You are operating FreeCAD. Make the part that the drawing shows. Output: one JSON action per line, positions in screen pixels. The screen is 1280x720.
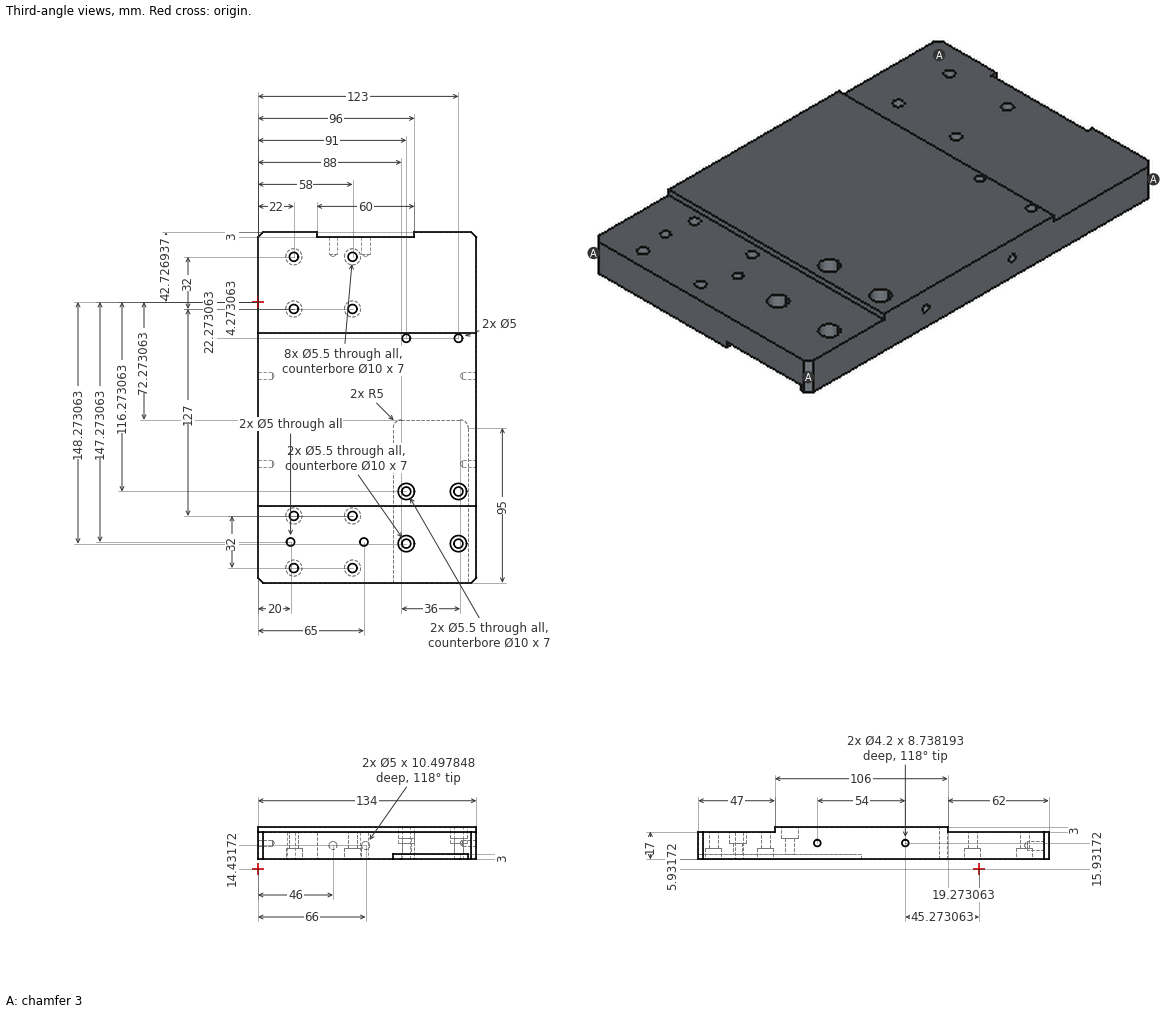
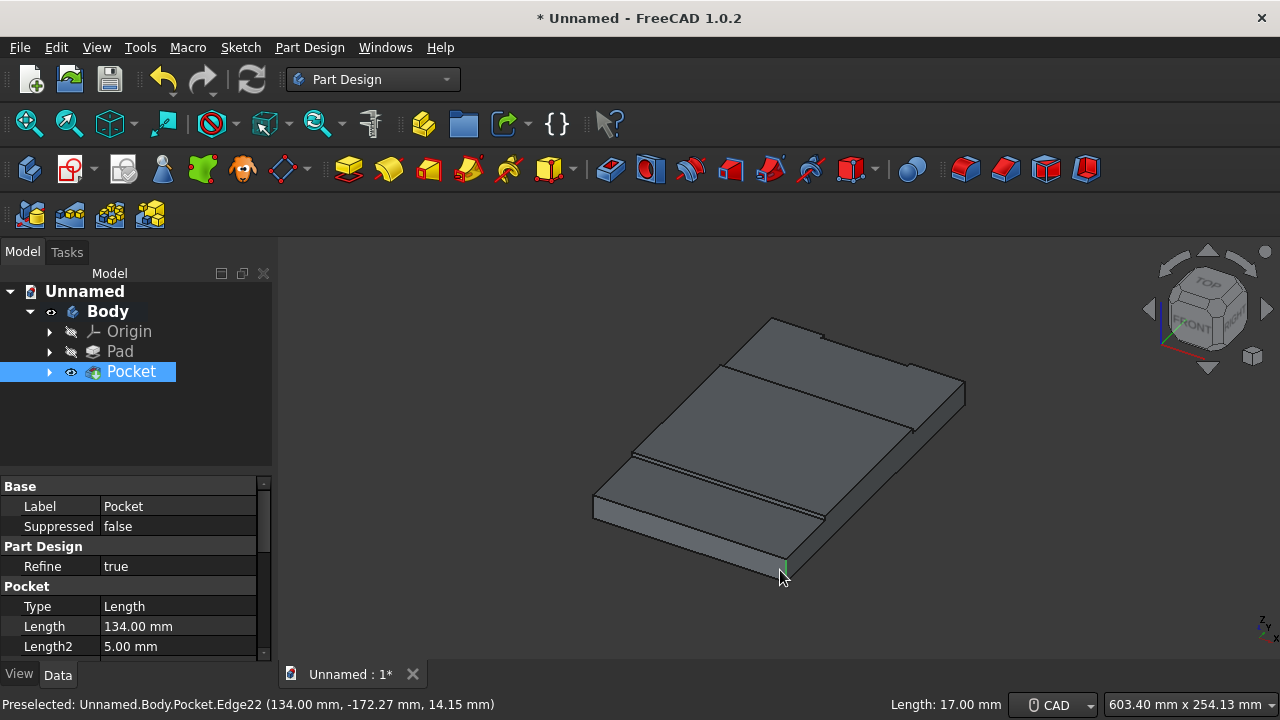
{"action": "key", "text": "0"}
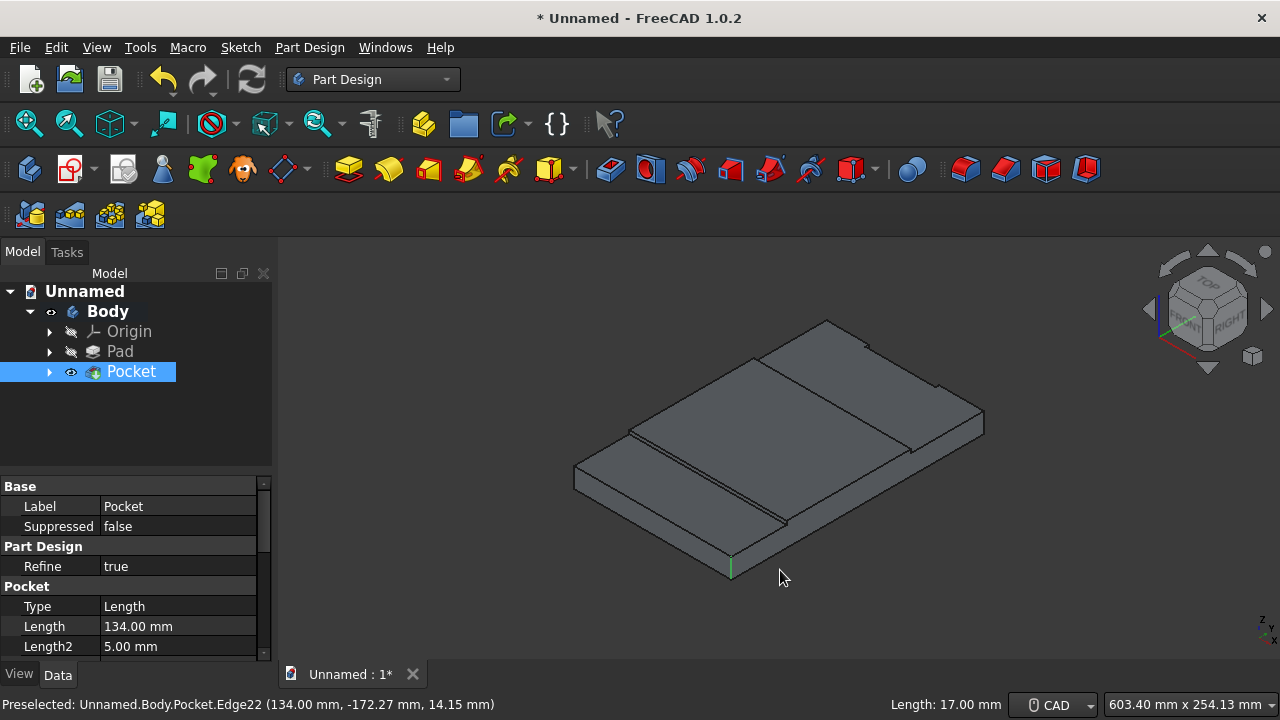
{"action": "key", "text": "2"}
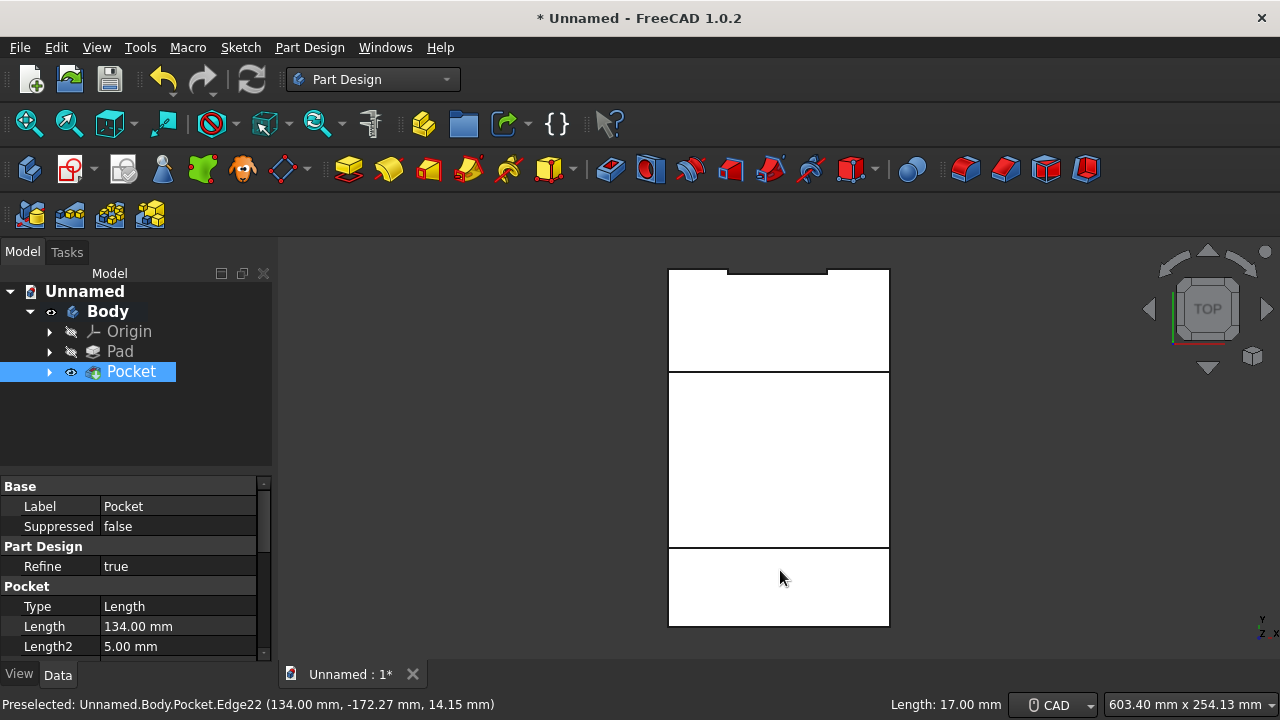
{"action": "key", "text": "1"}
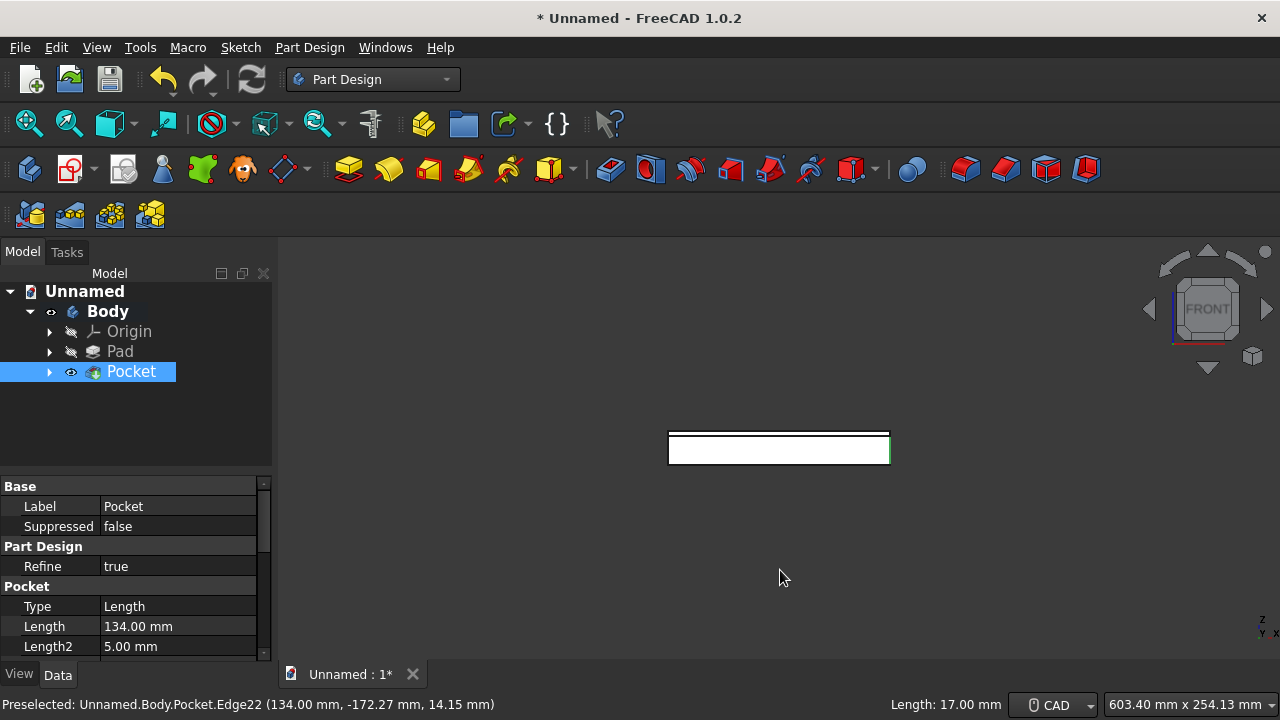
{"action": "left_click", "coordinate": [30, 124]}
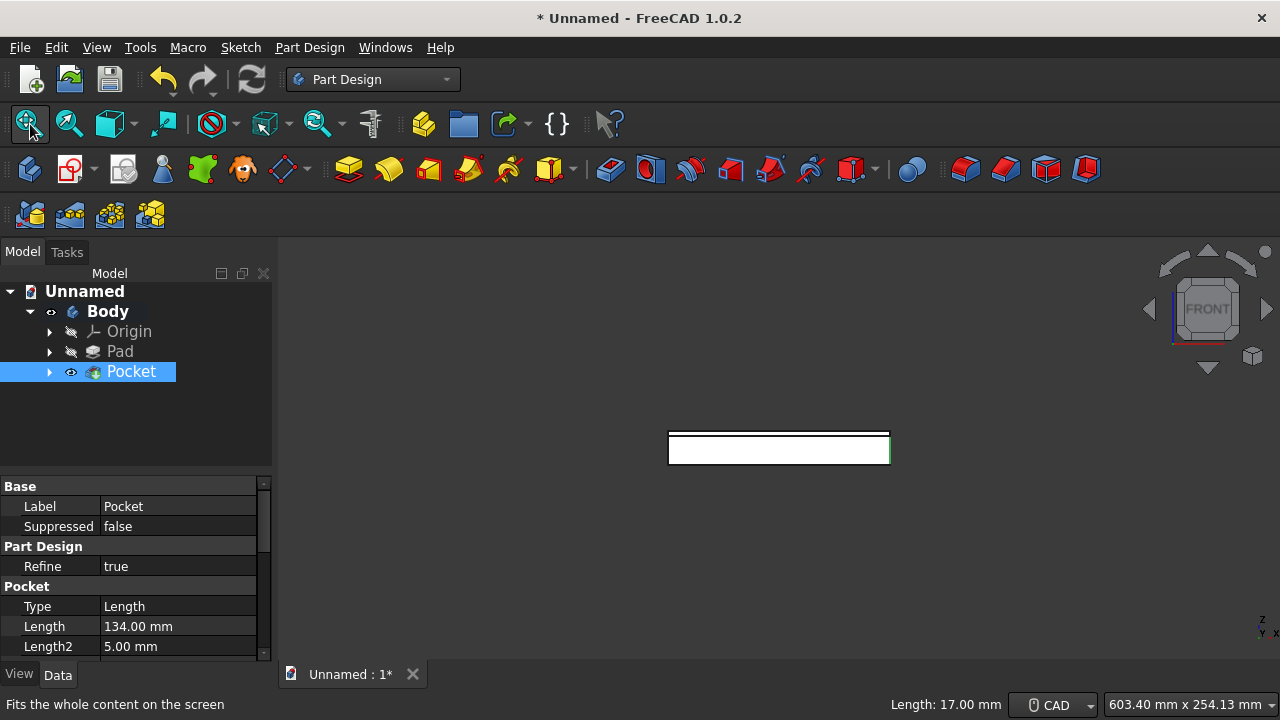
{"action": "left_click", "coordinate": [668, 449], "text": "ctrl"}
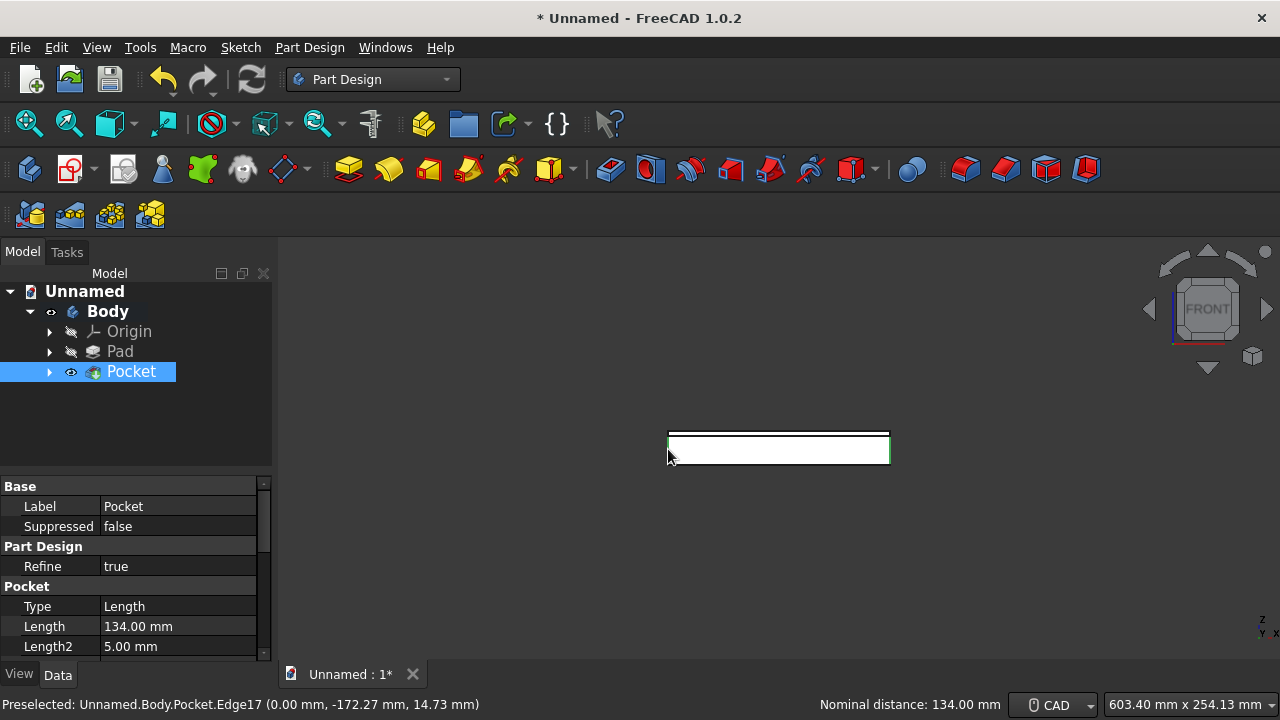
{"action": "key", "text": "3"}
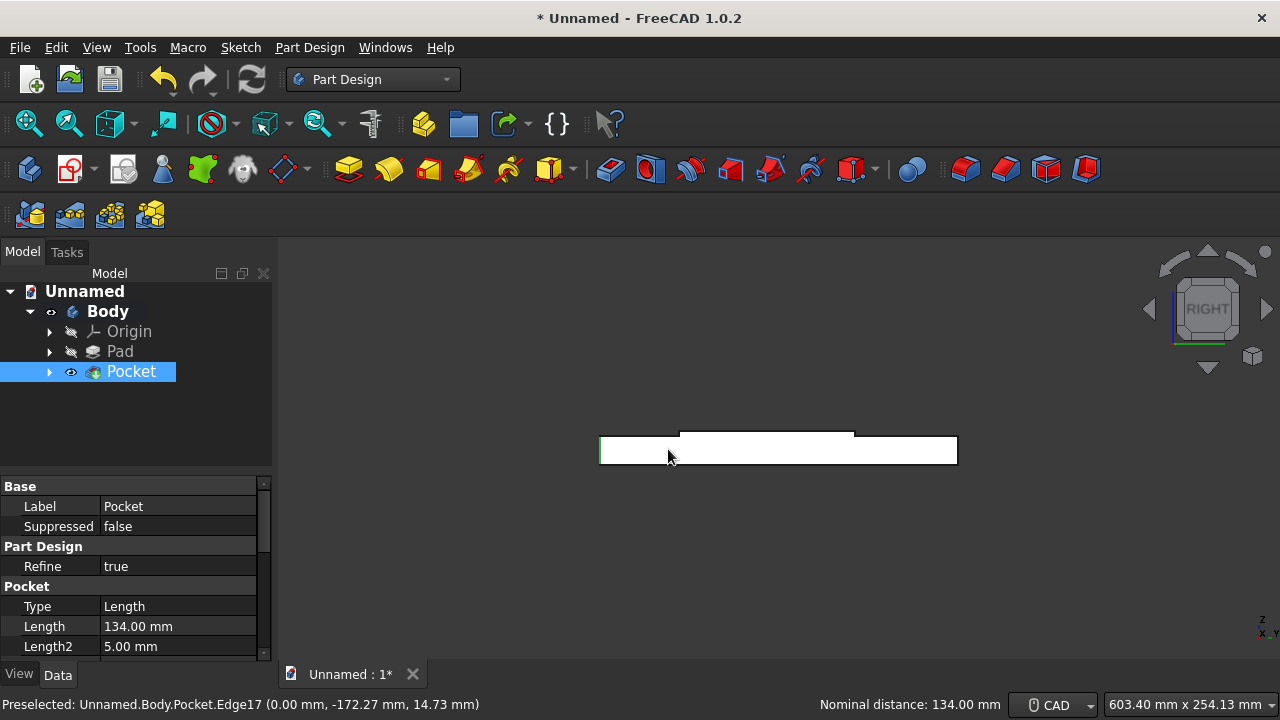
{"action": "left_click", "coordinate": [30, 124]}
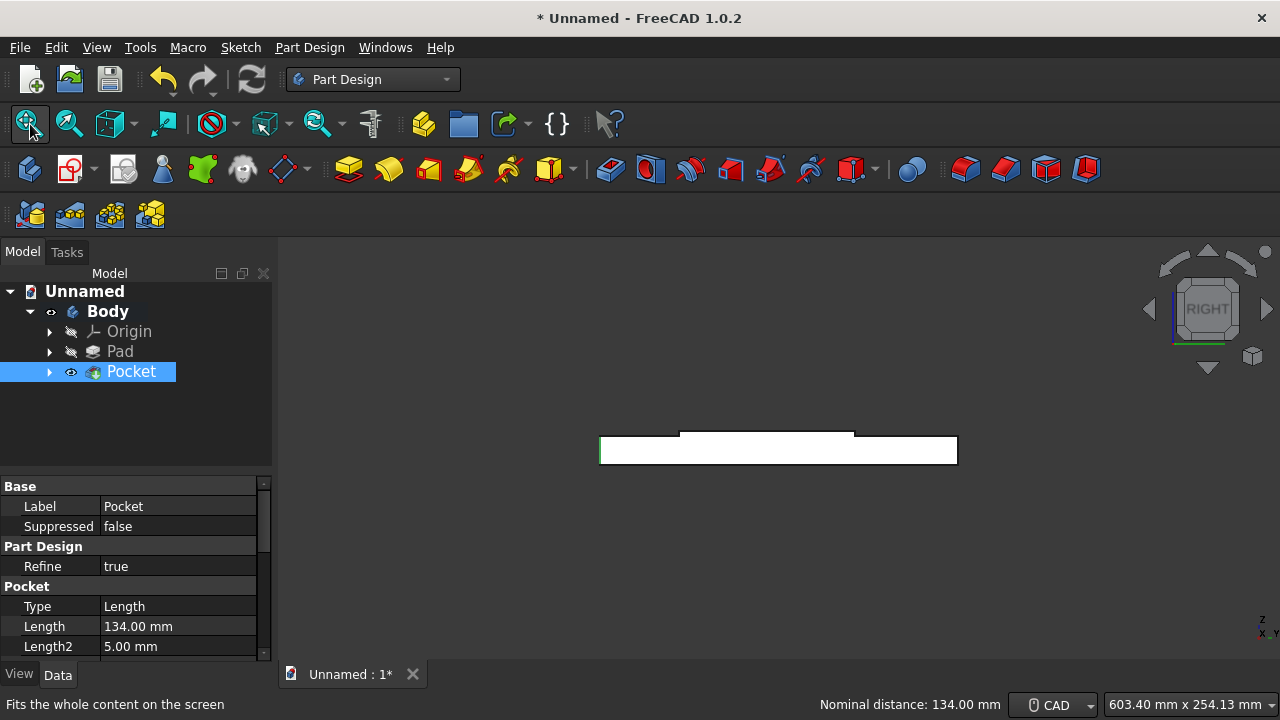
{"action": "left_click", "coordinate": [958, 449], "text": "ctrl"}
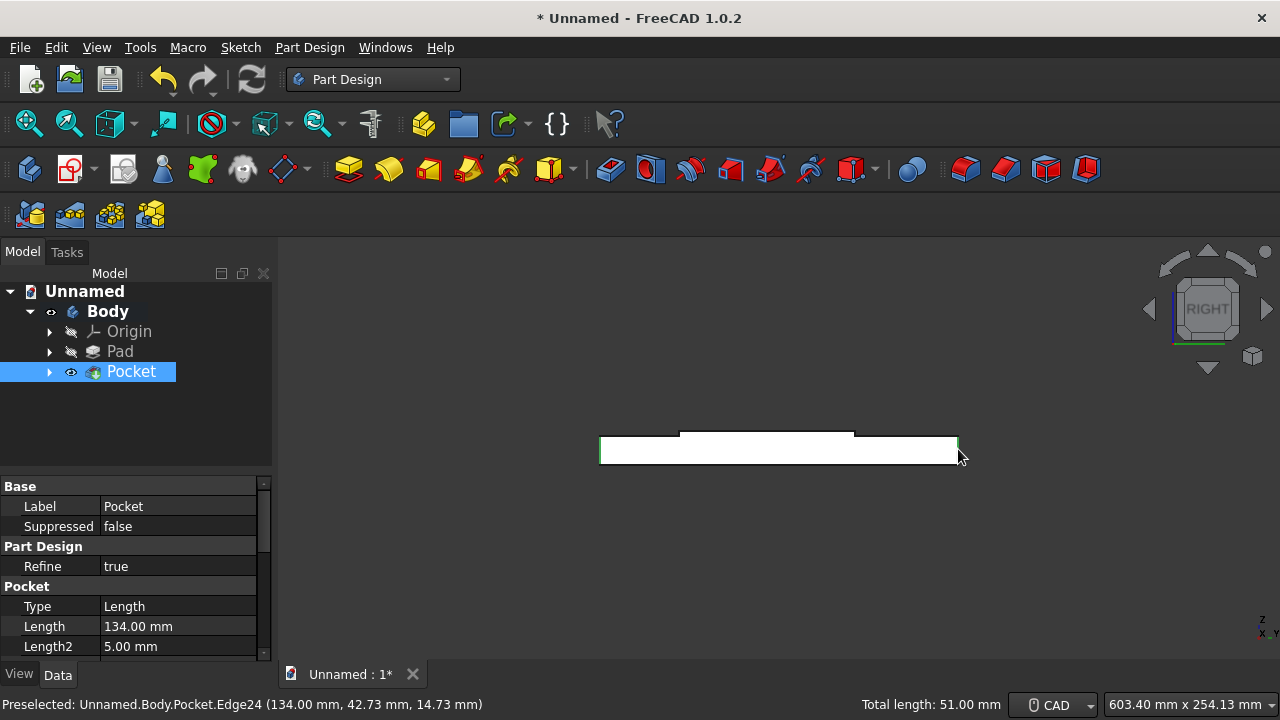
{"action": "key", "text": "5"}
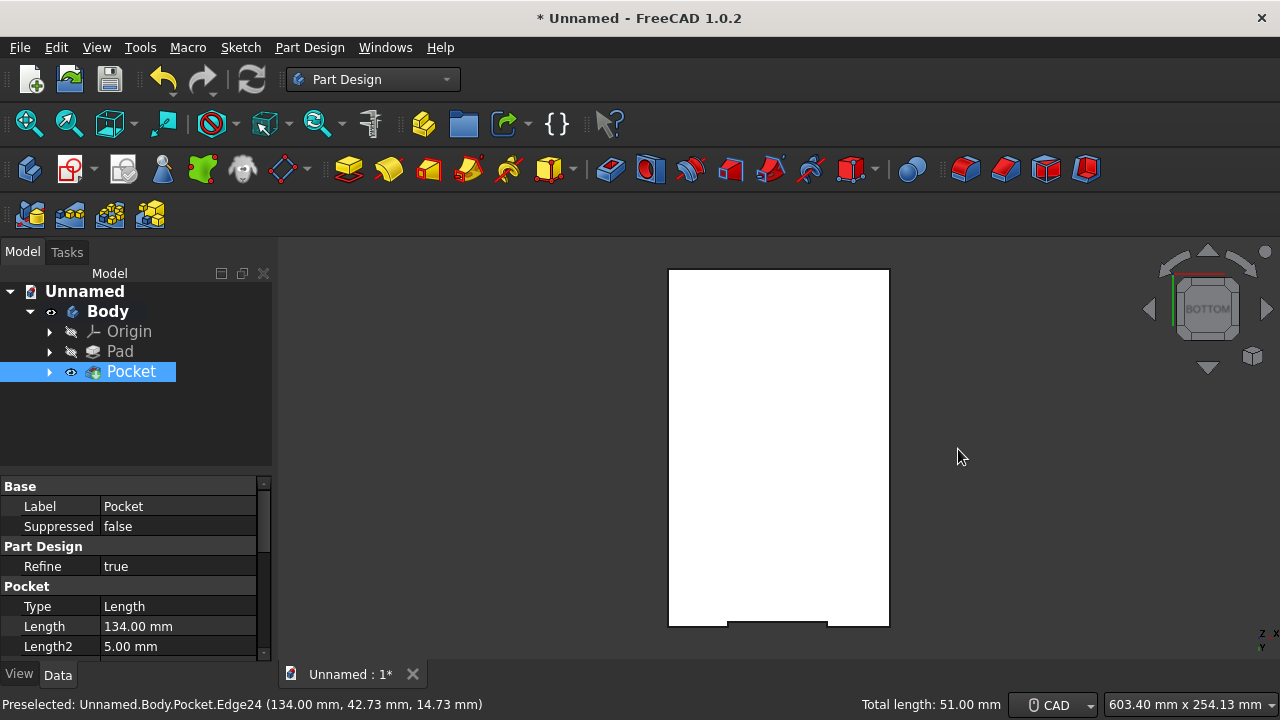
{"action": "key", "text": "4"}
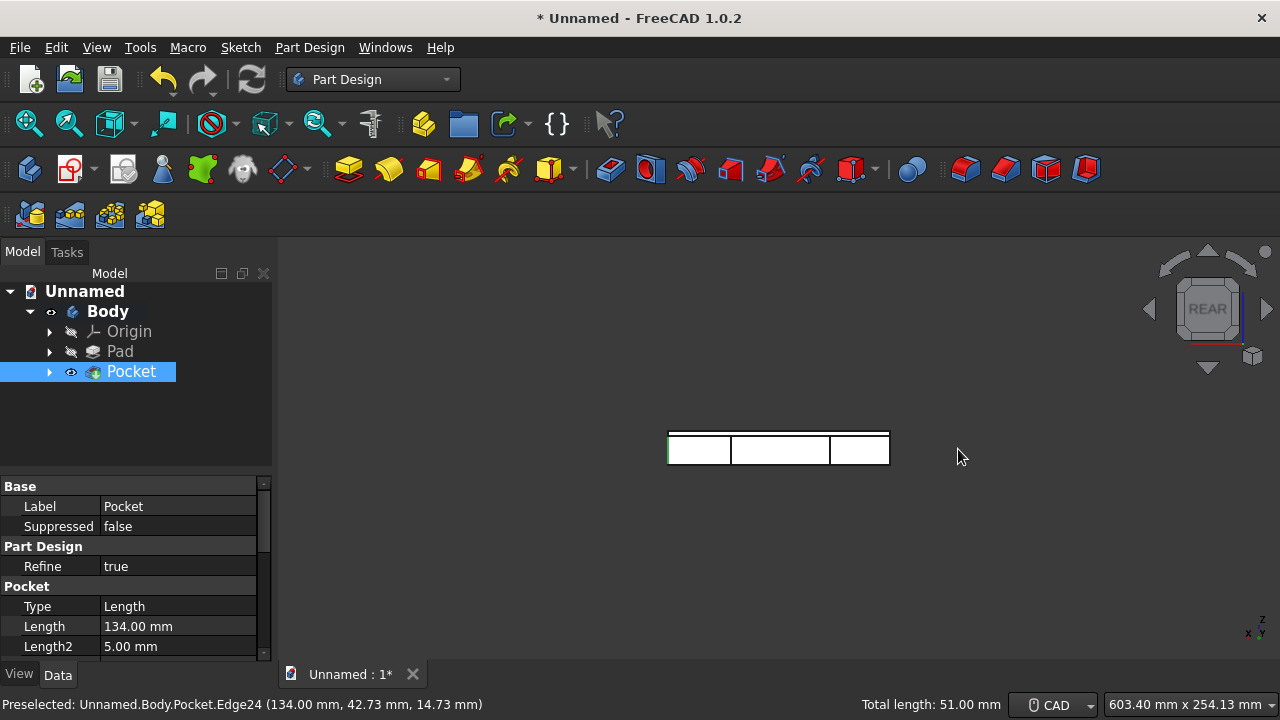
{"action": "left_click", "coordinate": [30, 124]}